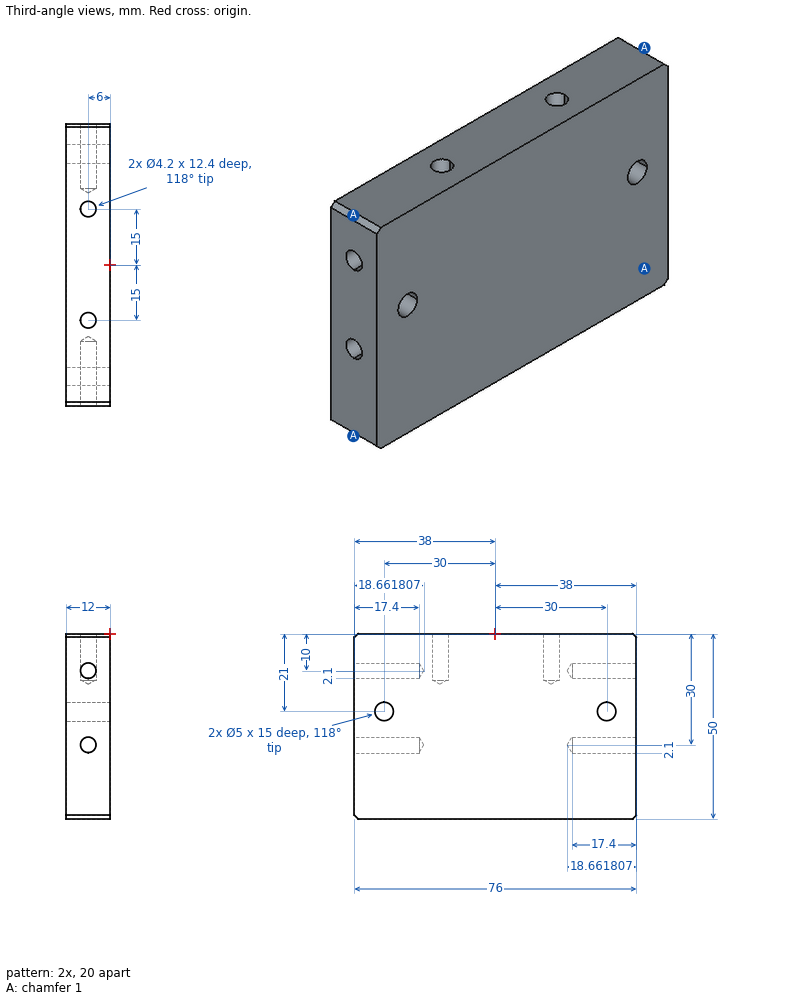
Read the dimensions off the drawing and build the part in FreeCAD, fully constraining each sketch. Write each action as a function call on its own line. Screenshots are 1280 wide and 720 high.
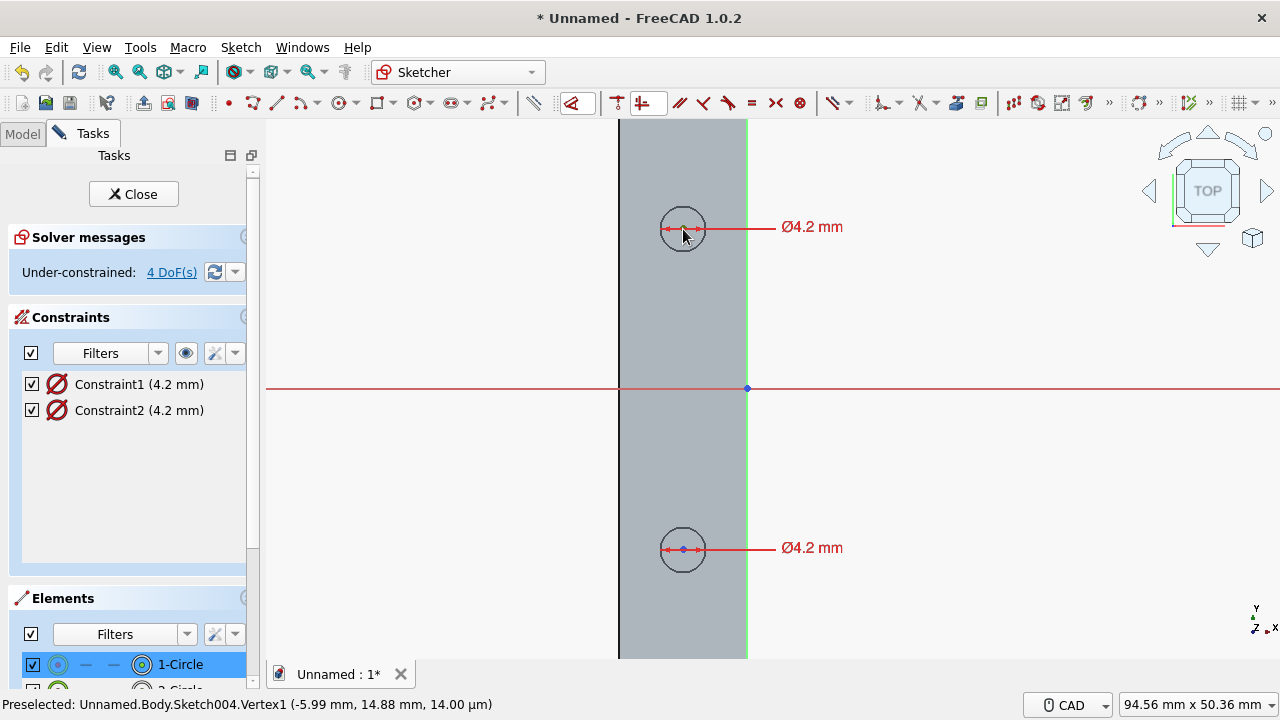
click(683, 550)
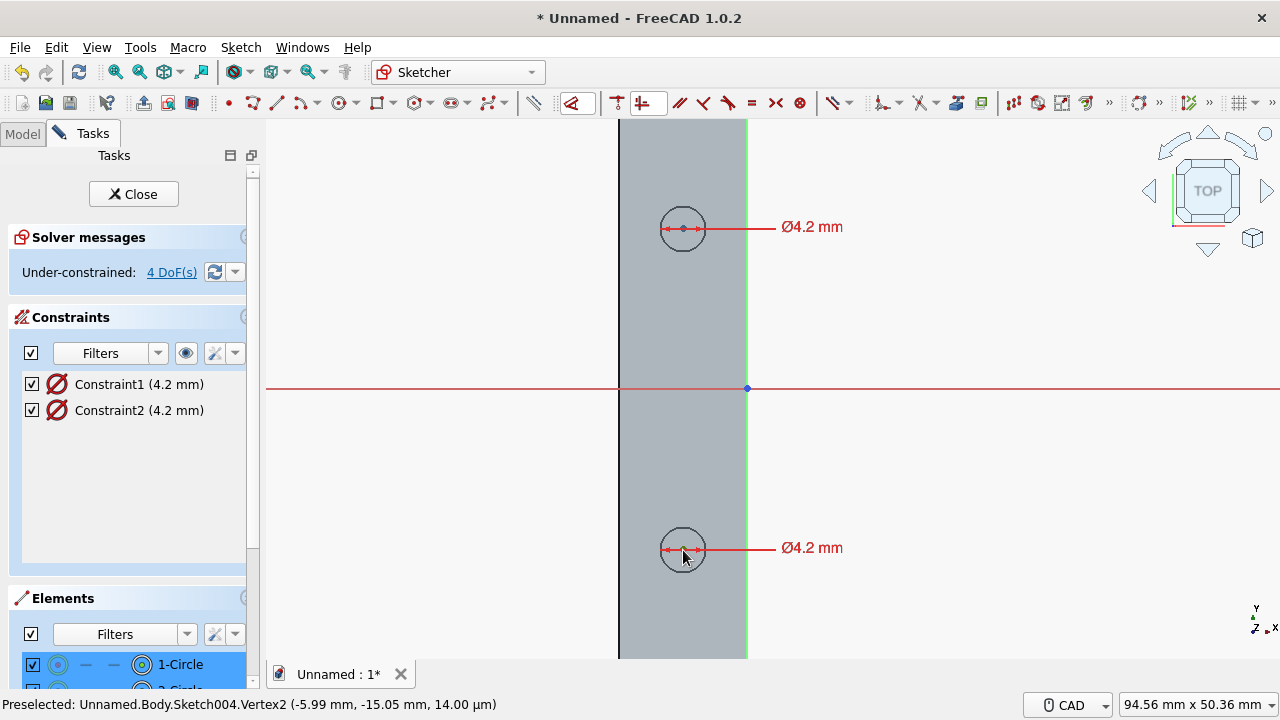
click(662, 104)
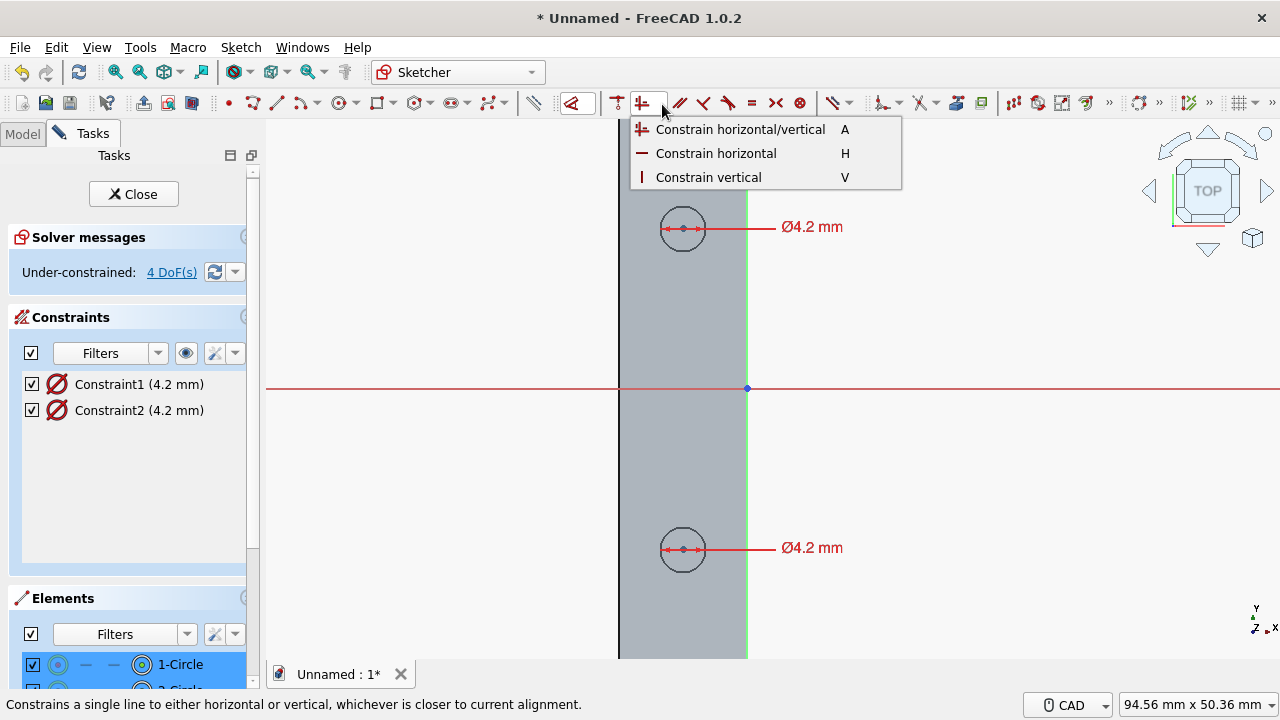
click(766, 177)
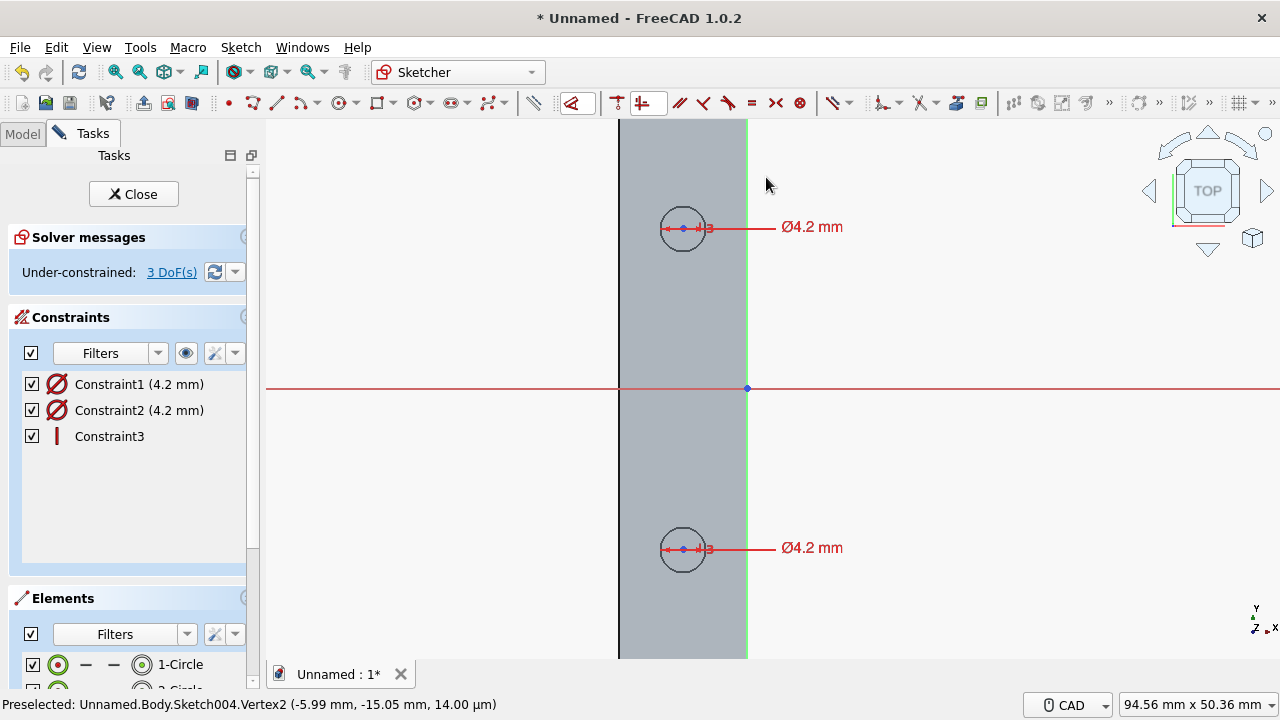
click(683, 229)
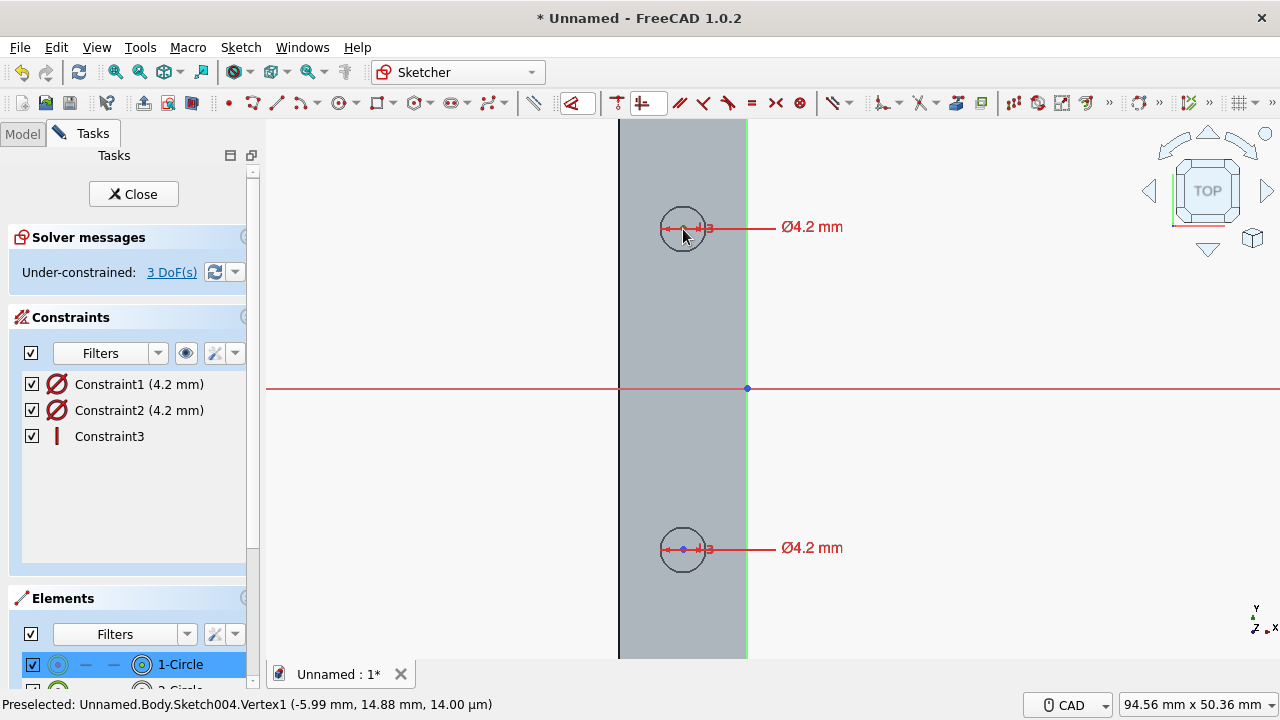
key(l)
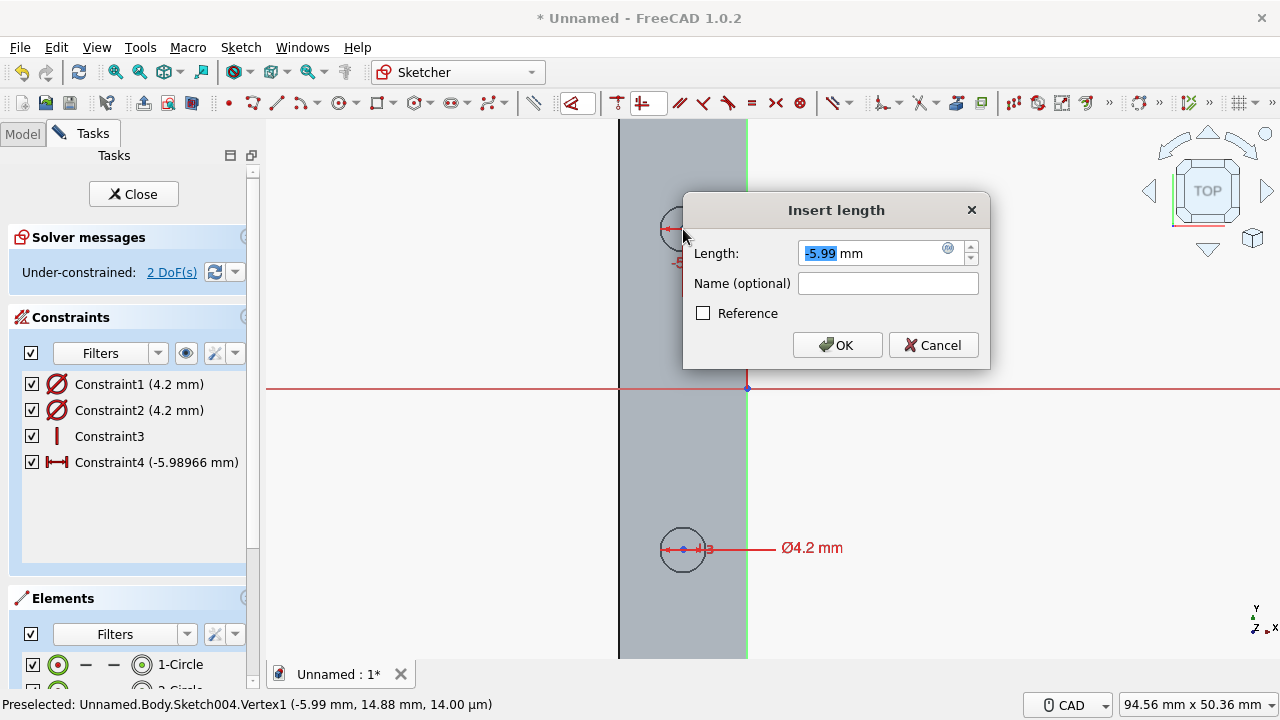
text(-6)
key(Return)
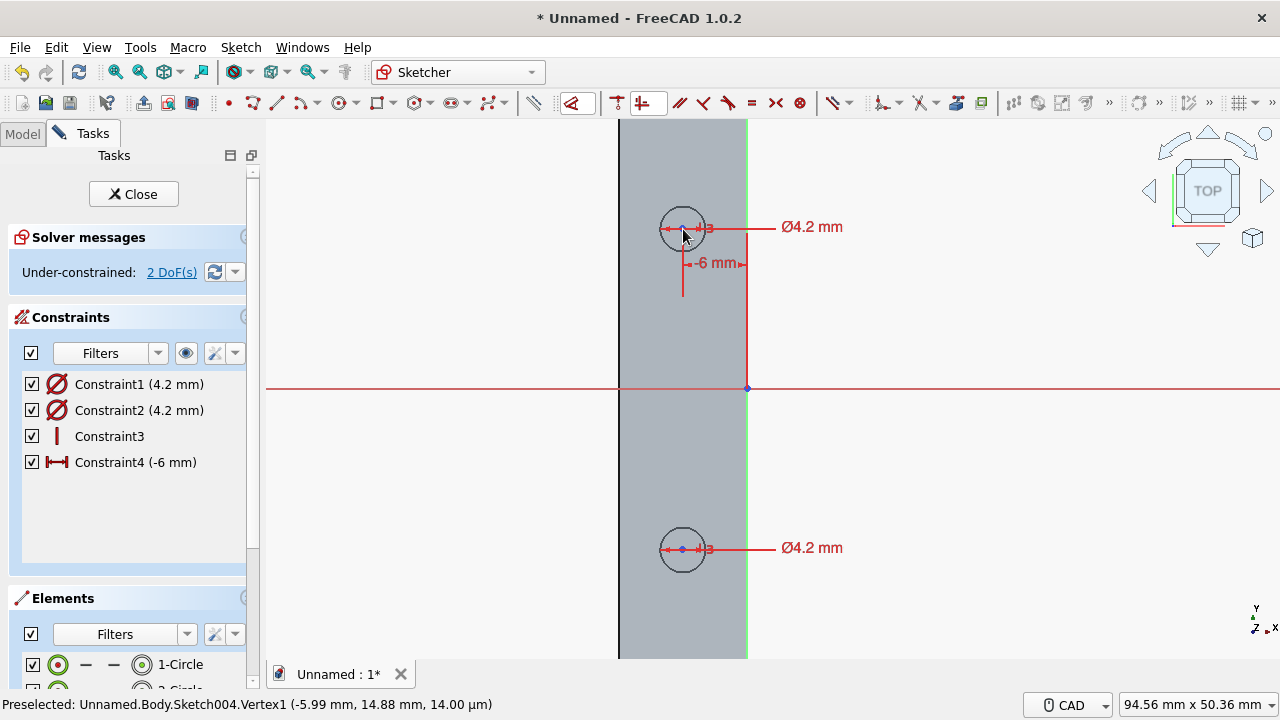
click(683, 229)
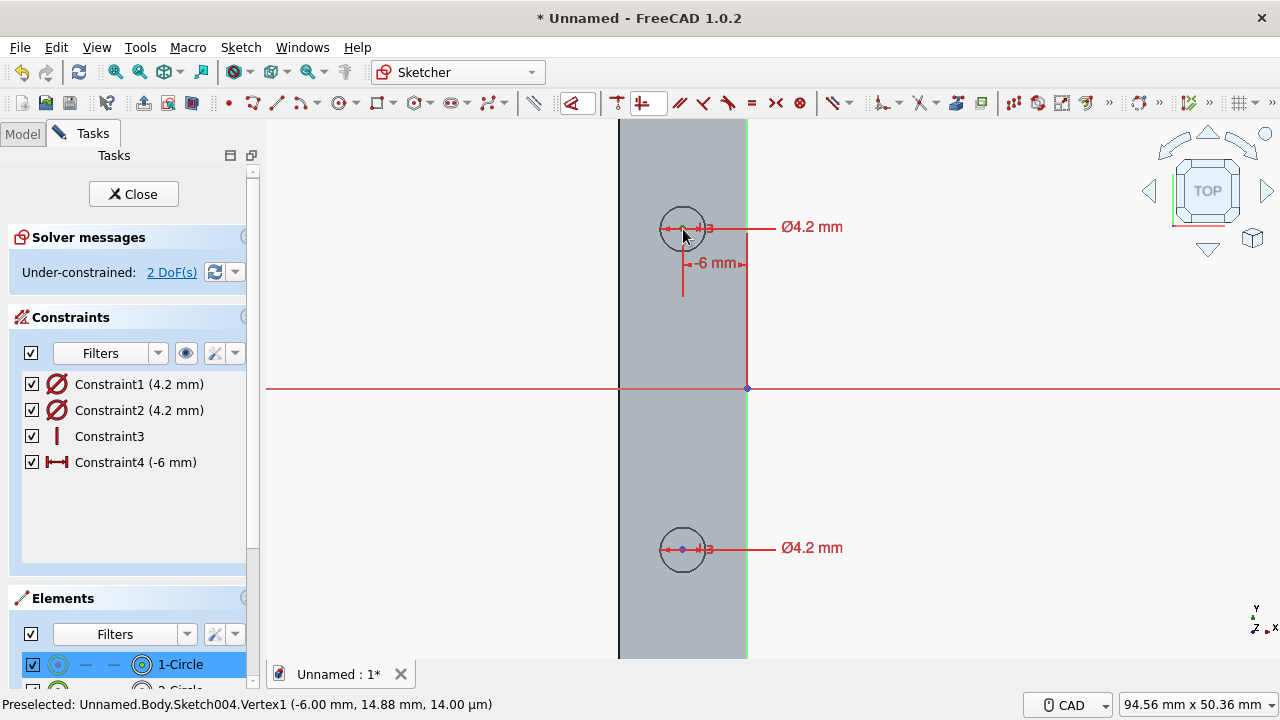
key(i)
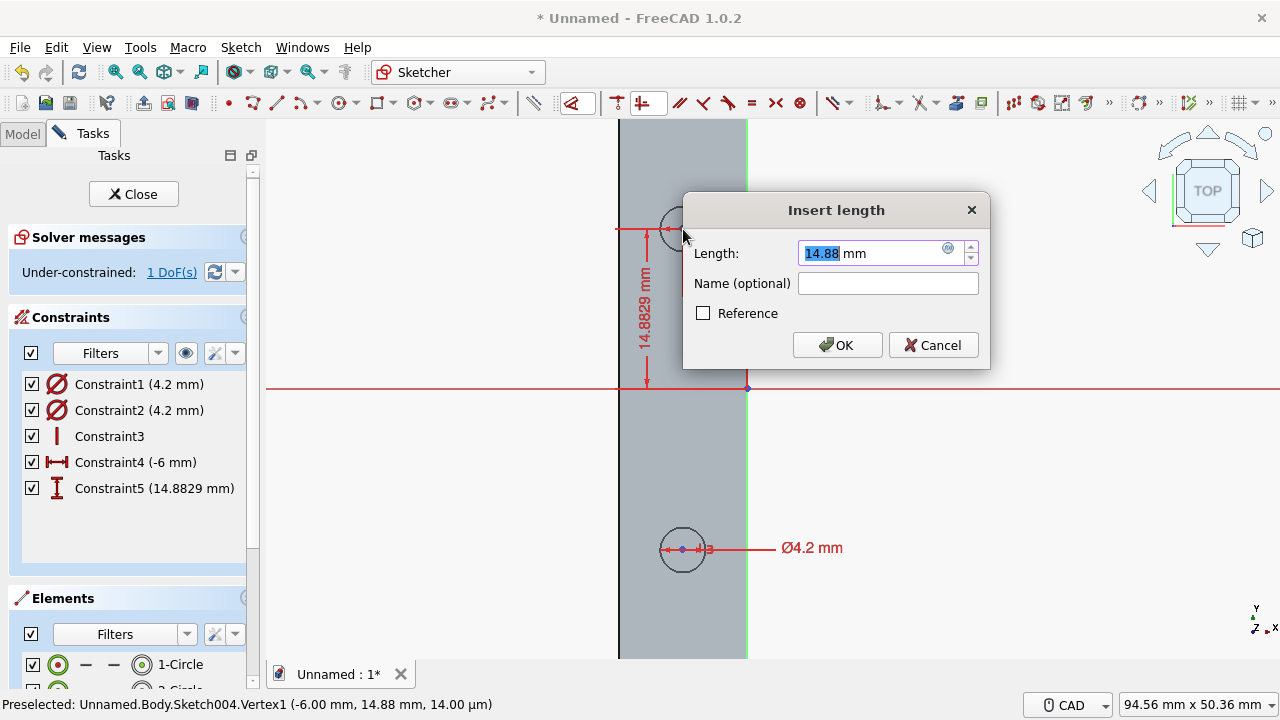
text(15)
key(Return)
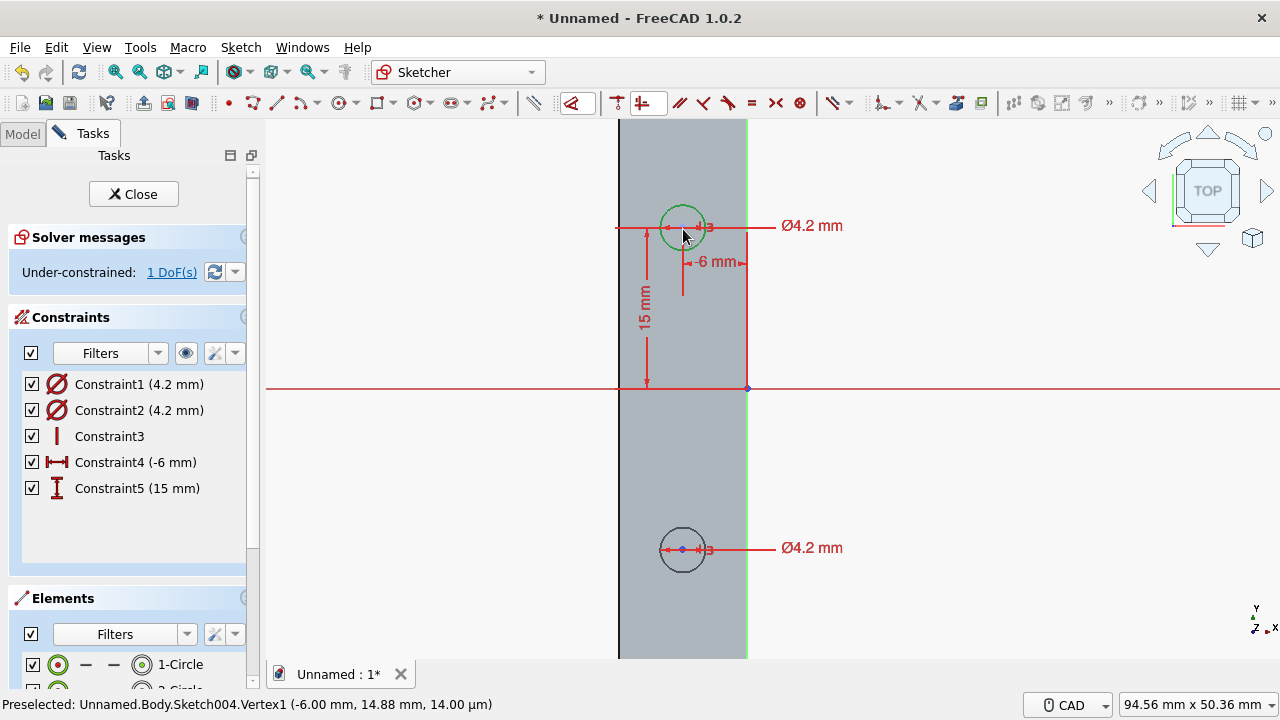
click(683, 550)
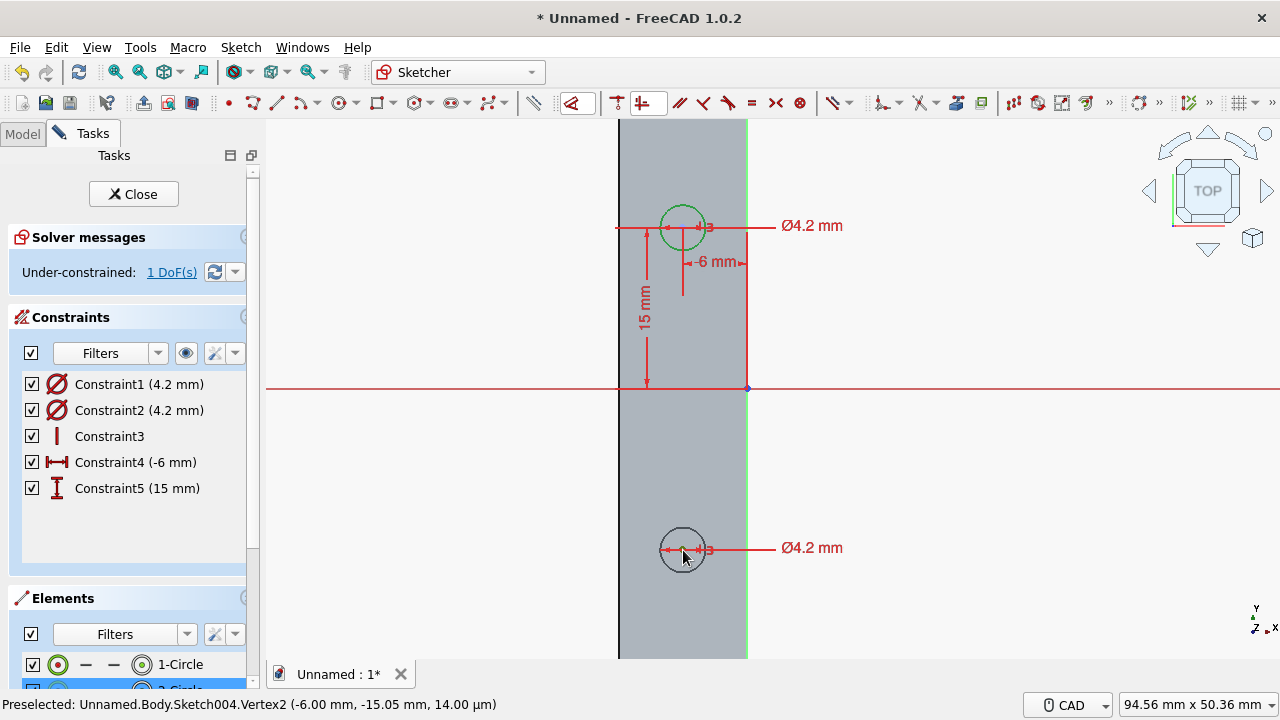
click(590, 104)